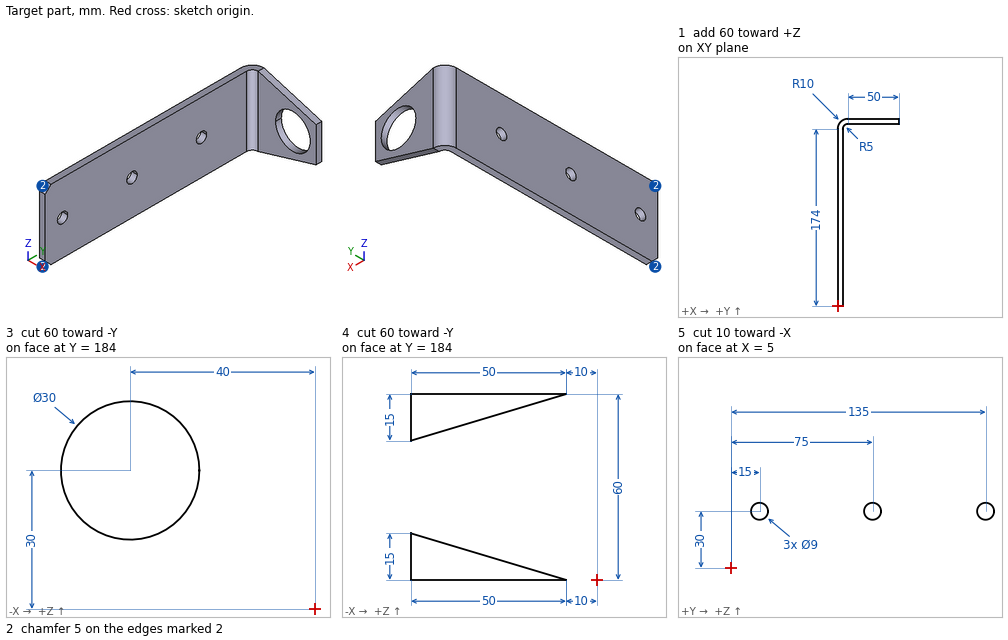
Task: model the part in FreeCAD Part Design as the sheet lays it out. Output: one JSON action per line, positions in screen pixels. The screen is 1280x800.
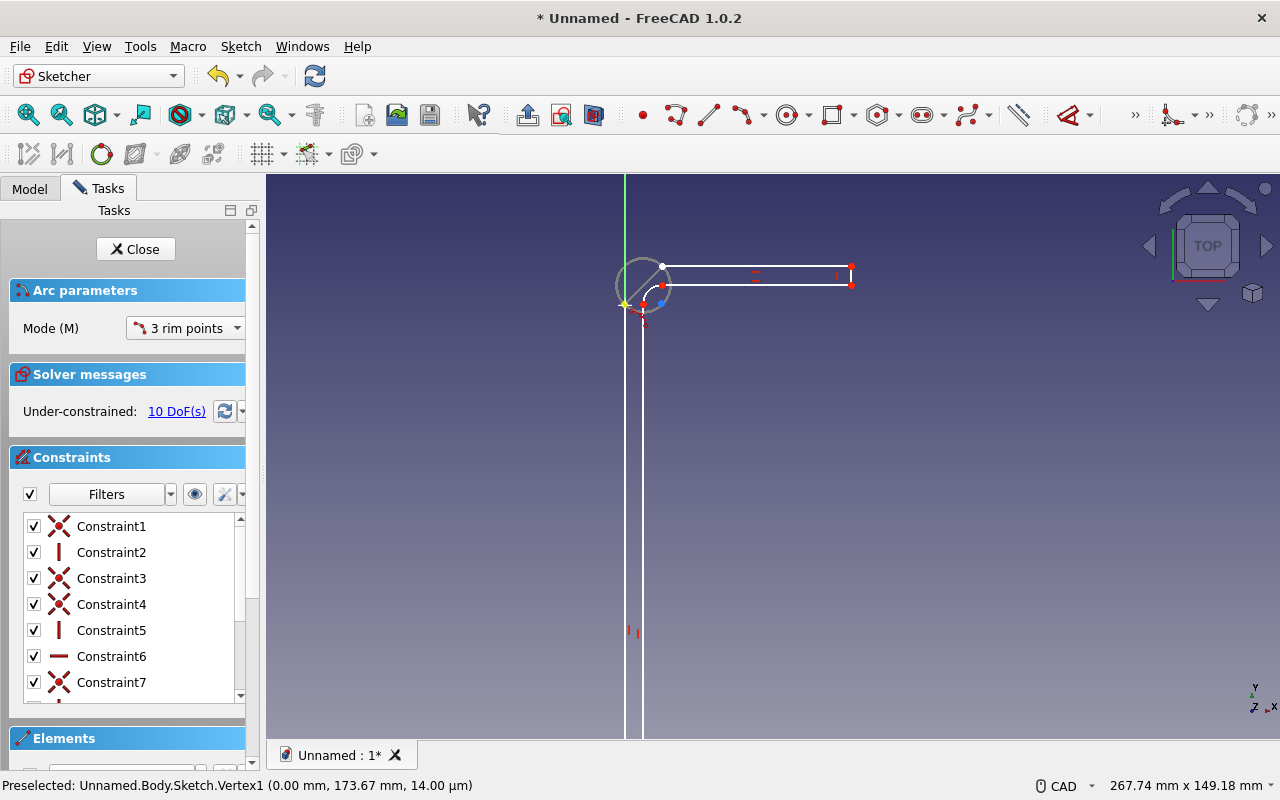
{"action": "scroll", "coordinate": [636, 277], "scroll_direction": "up", "scroll_amount": 2}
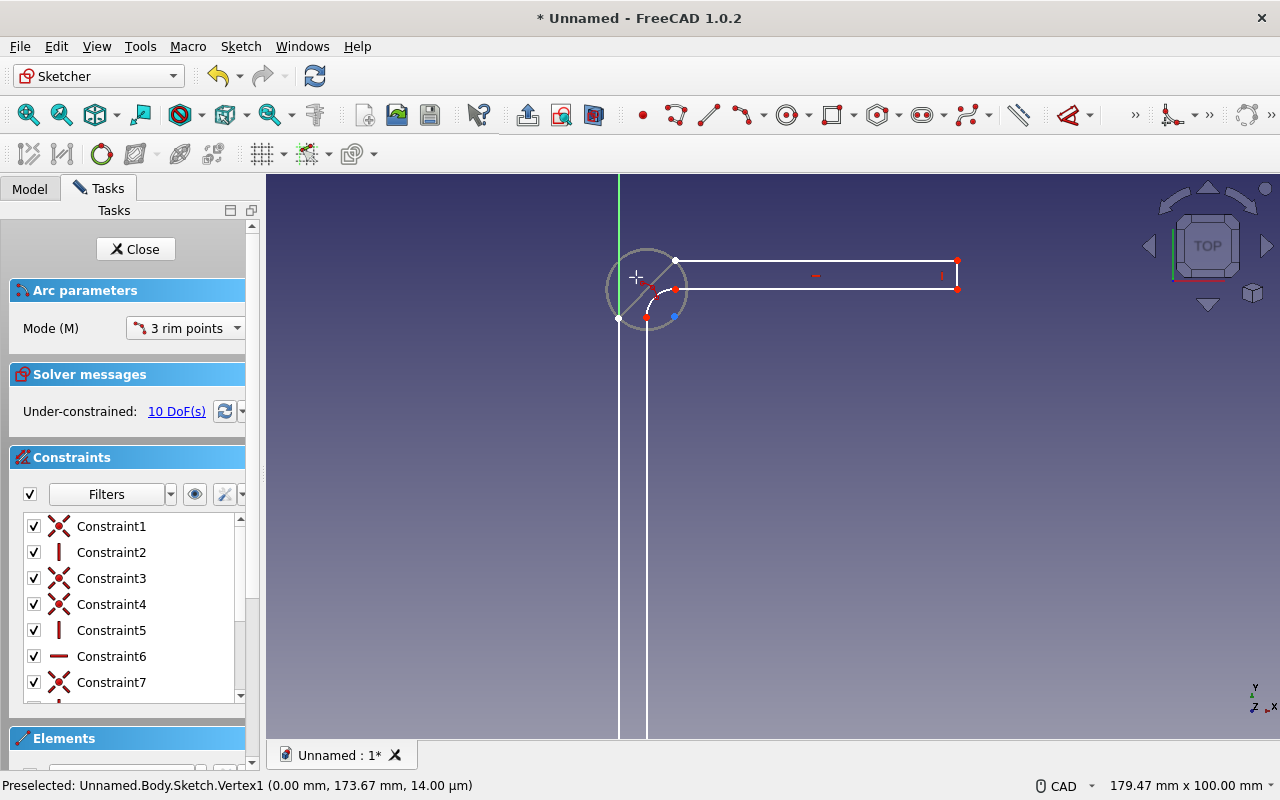
{"action": "left_click", "coordinate": [635, 276]}
{"action": "key", "text": "Escape"}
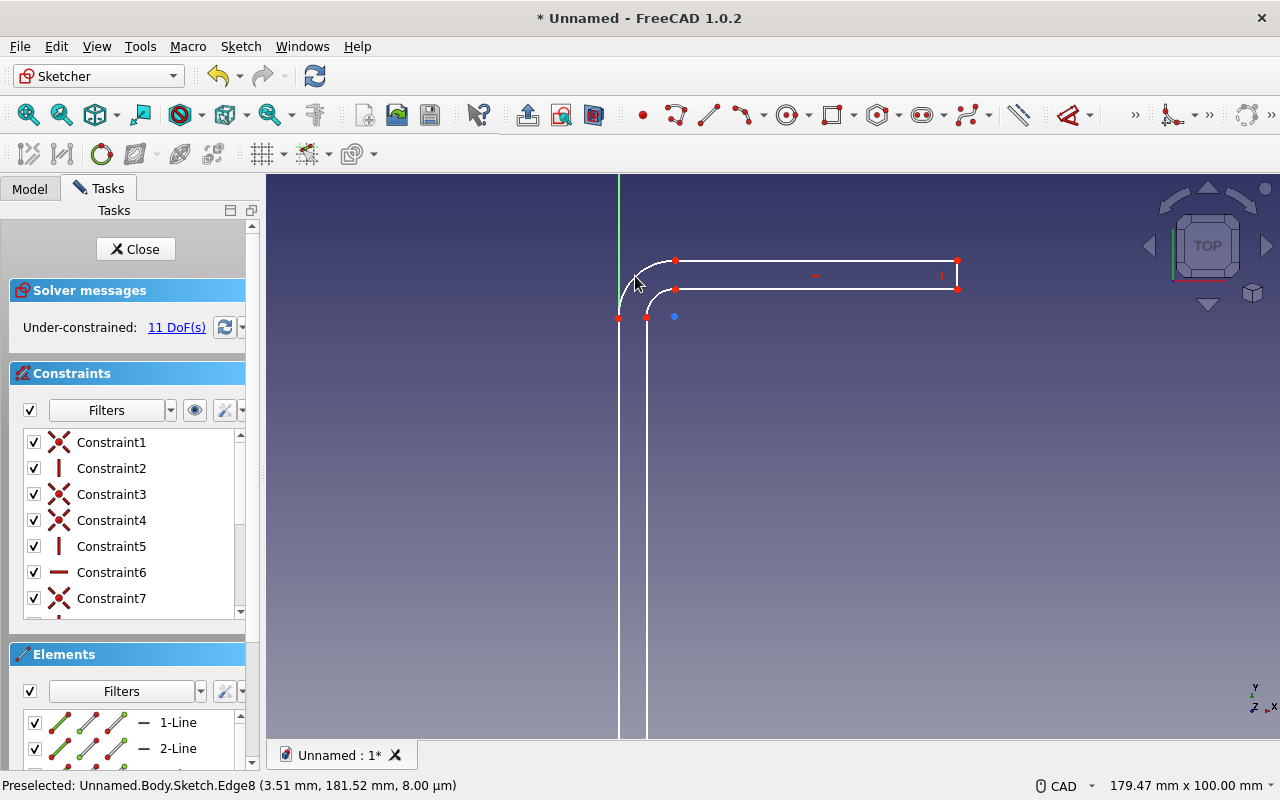
{"action": "left_click", "coordinate": [619, 612]}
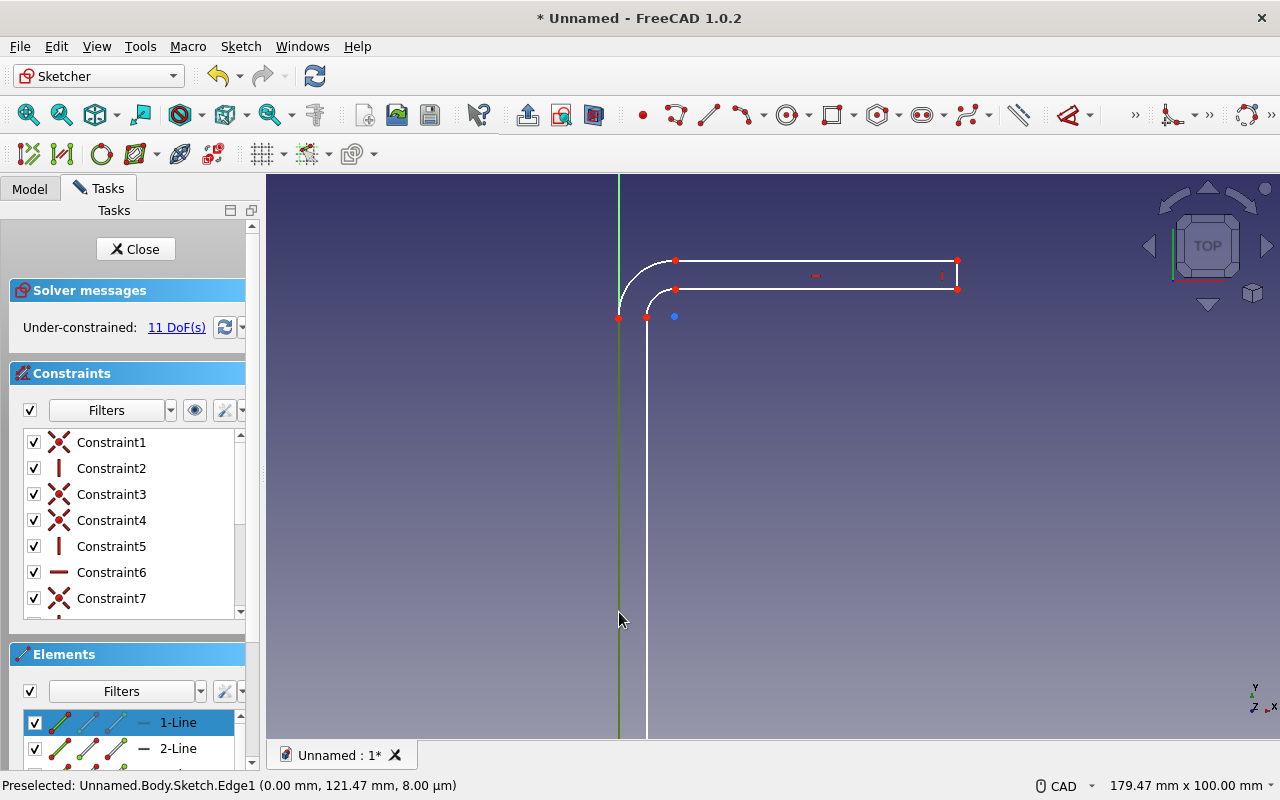
{"action": "left_click", "coordinate": [649, 267]}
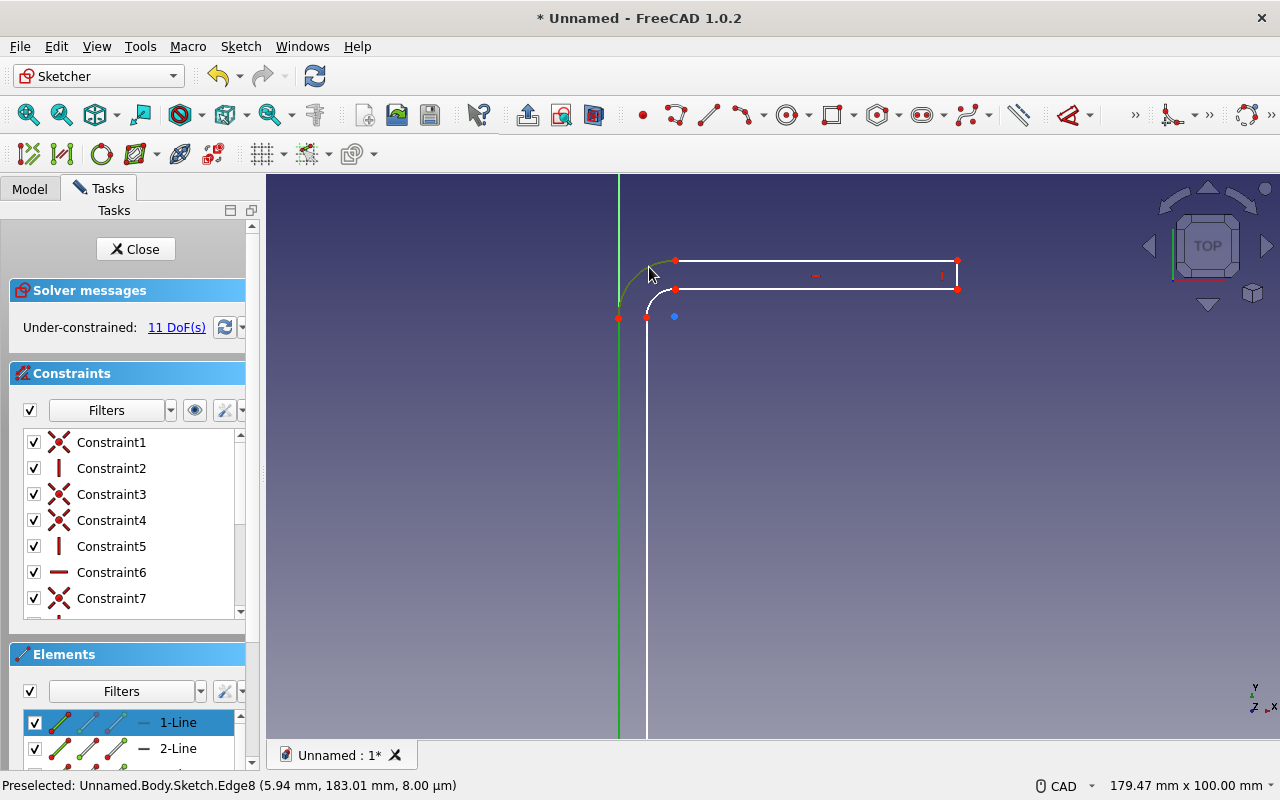
{"action": "key", "text": "t"}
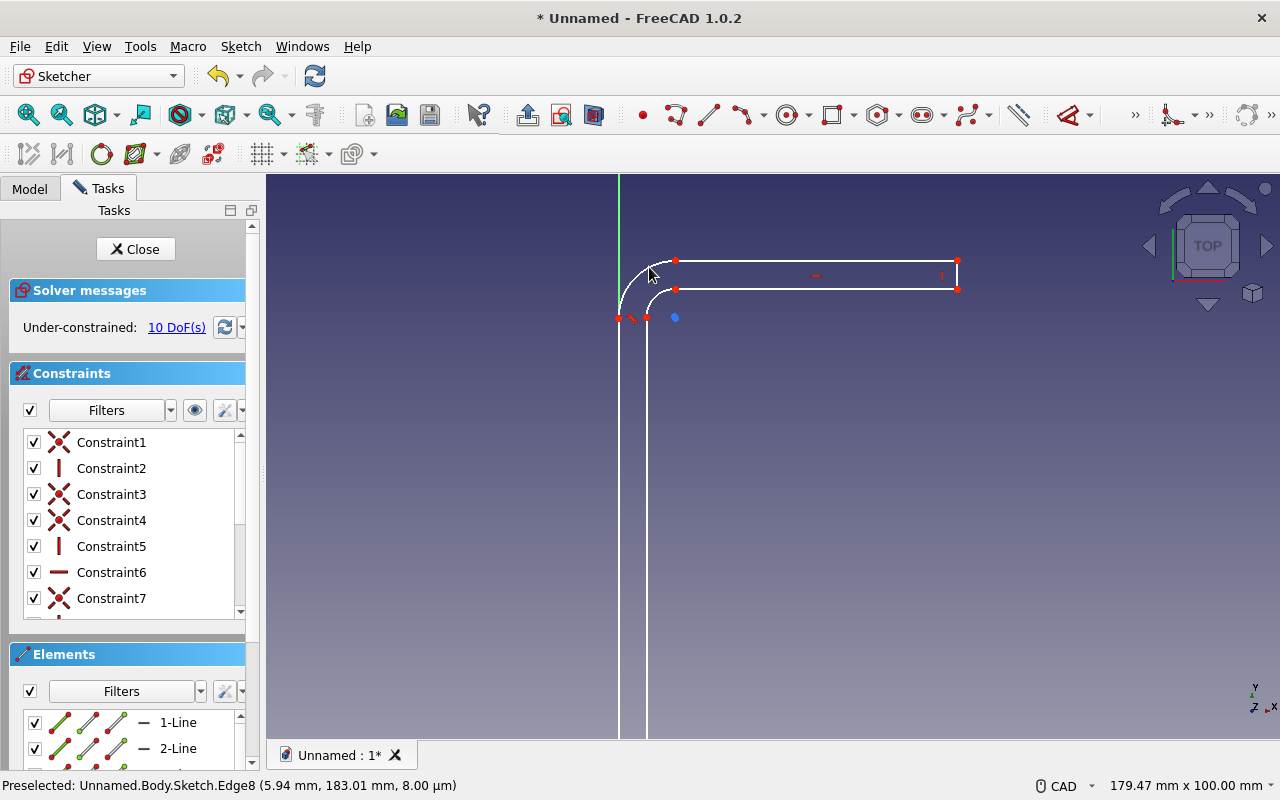
{"action": "left_click", "coordinate": [647, 608]}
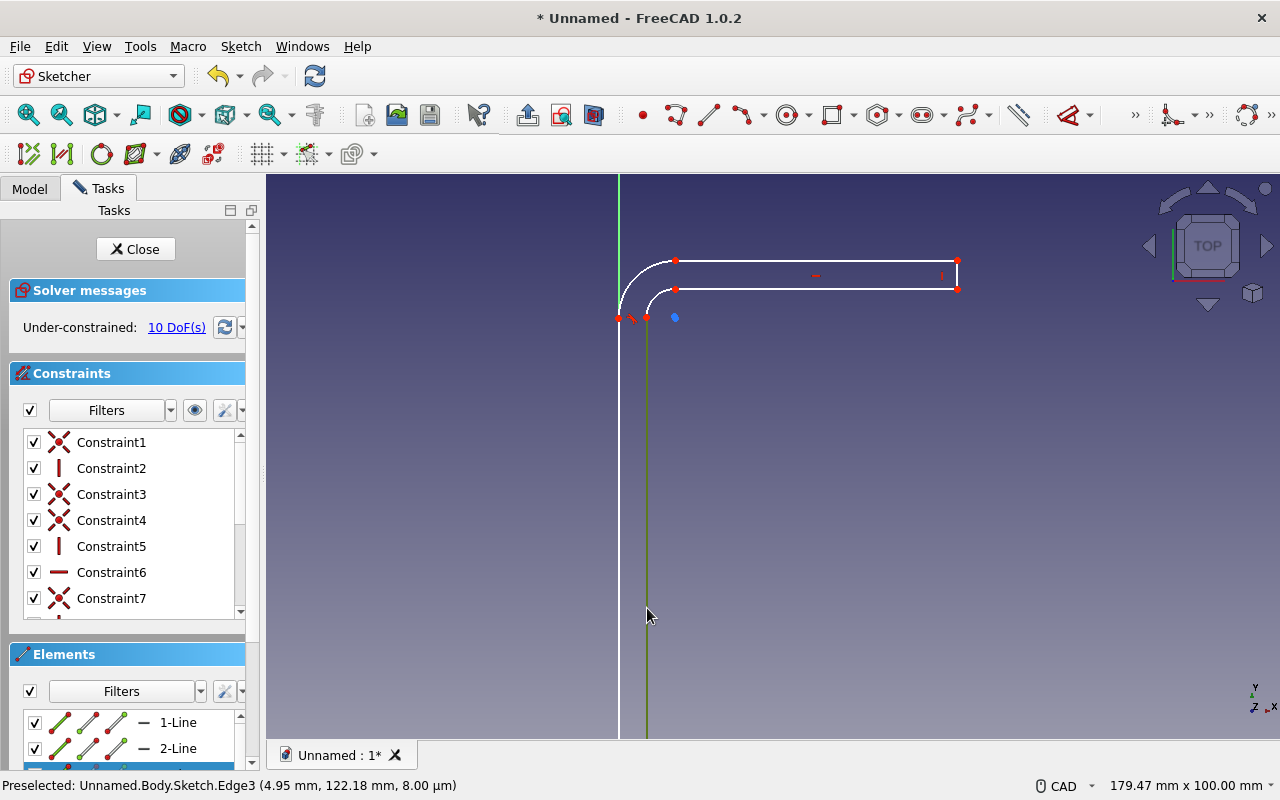
{"action": "left_click", "coordinate": [662, 292]}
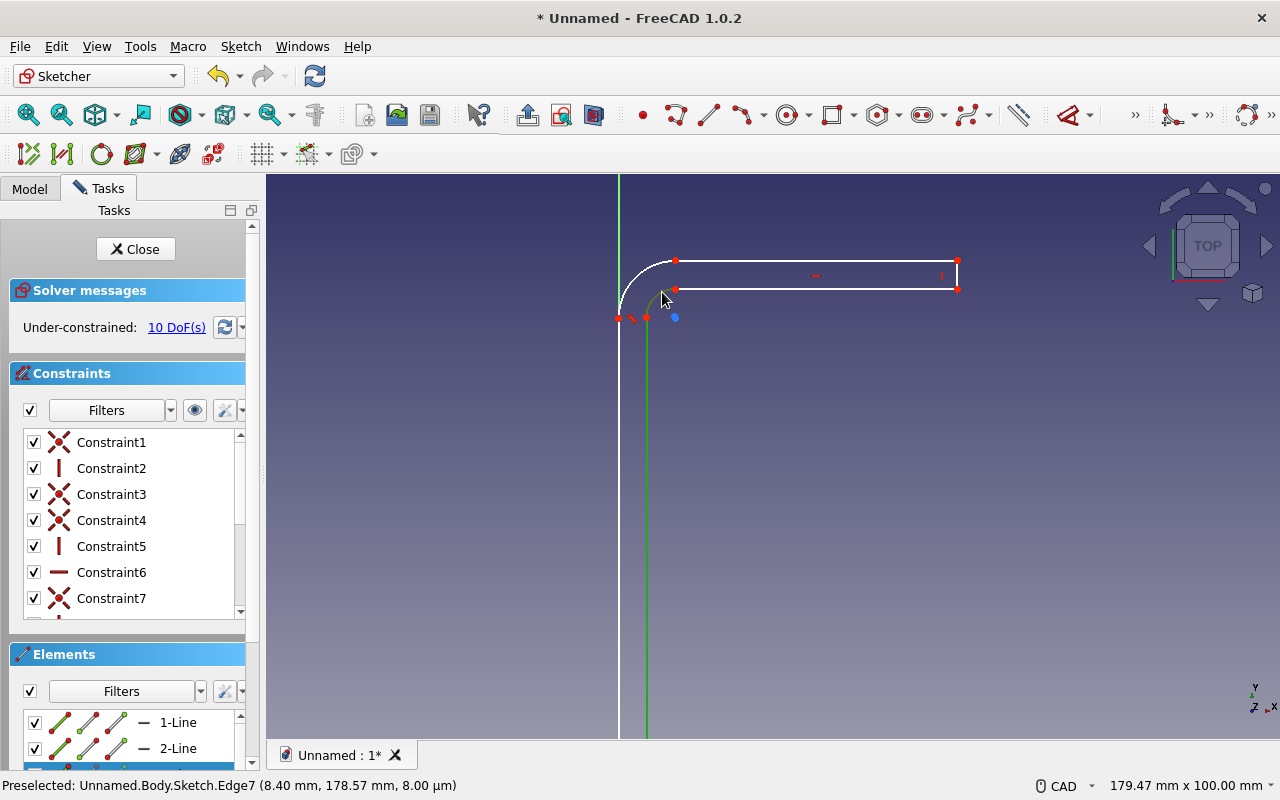
{"action": "key", "text": "t"}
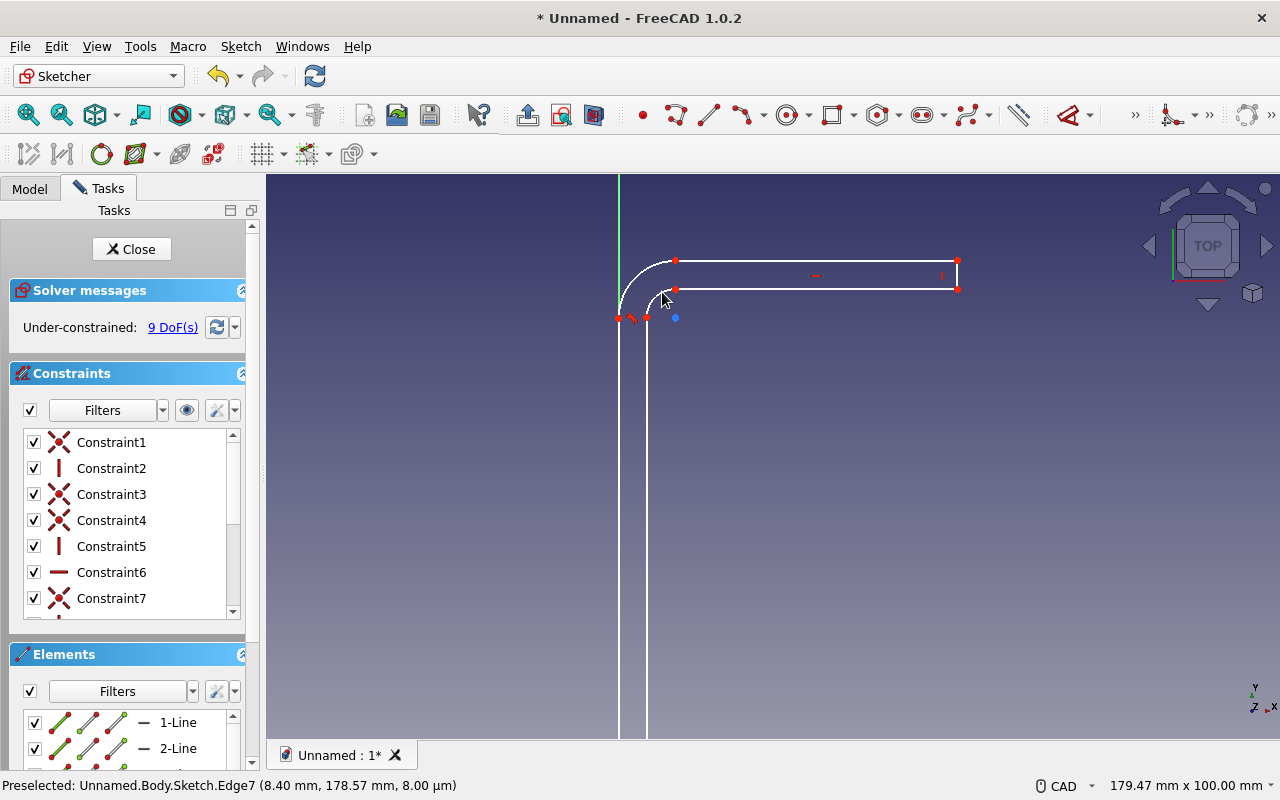
{"action": "left_click", "coordinate": [760, 289]}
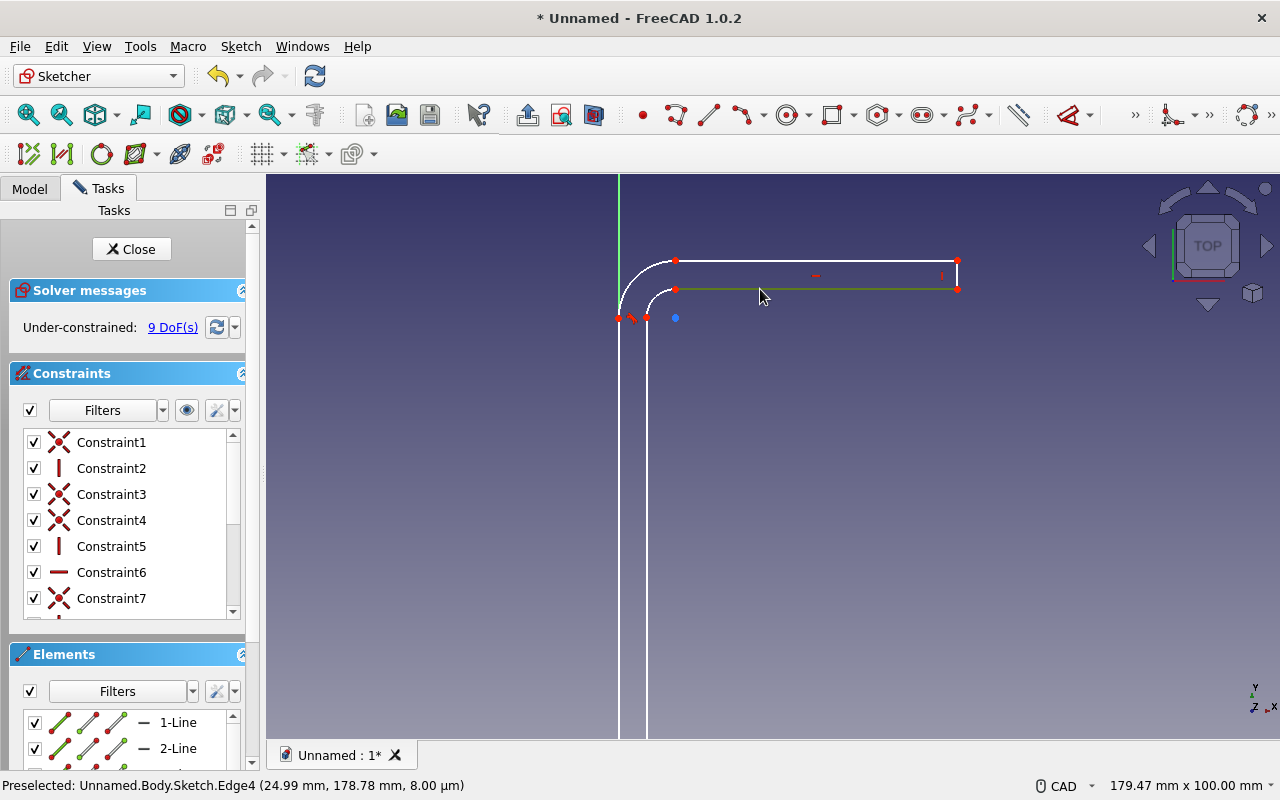
{"action": "left_click", "coordinate": [662, 292]}